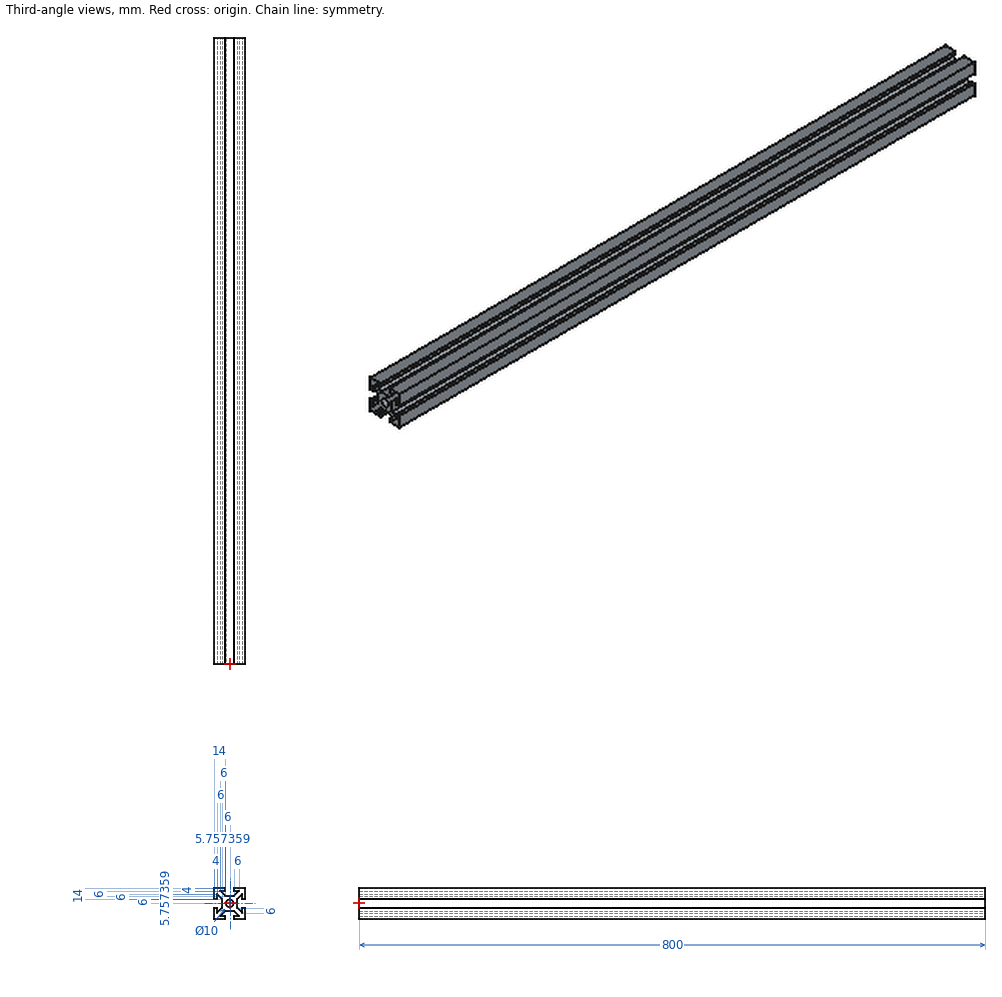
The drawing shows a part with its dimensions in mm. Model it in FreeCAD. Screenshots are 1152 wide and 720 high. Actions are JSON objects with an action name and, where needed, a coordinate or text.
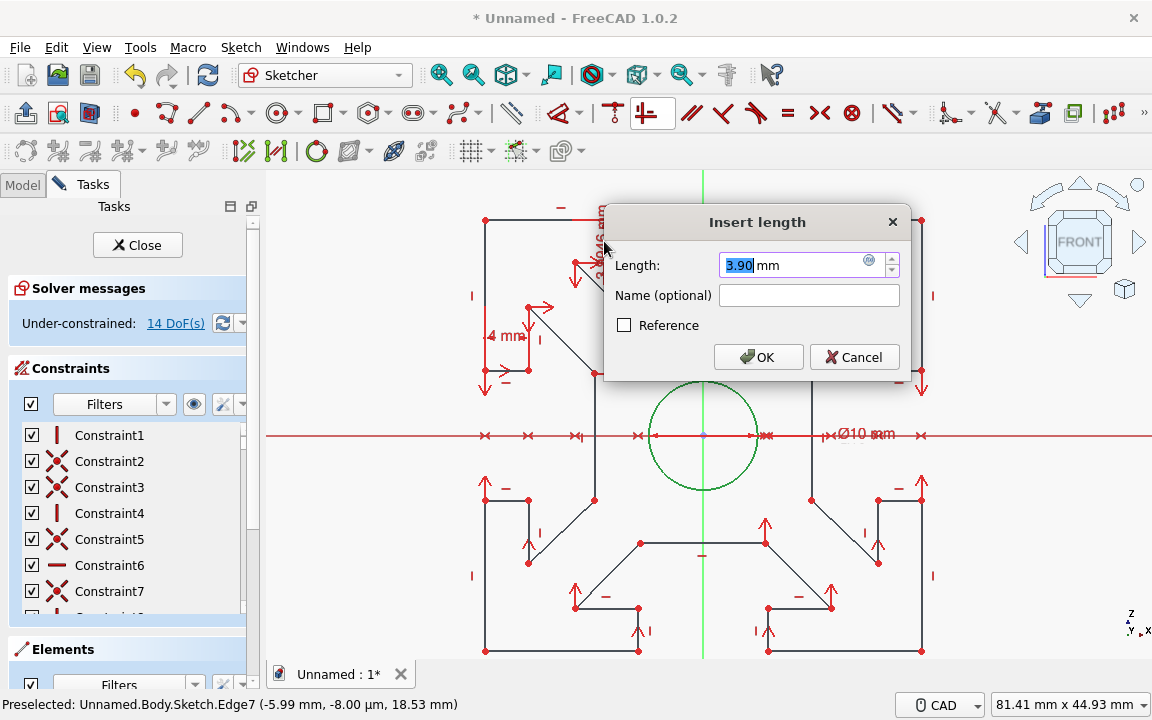
{"action": "type", "text": "4"}
{"action": "key", "text": "Return"}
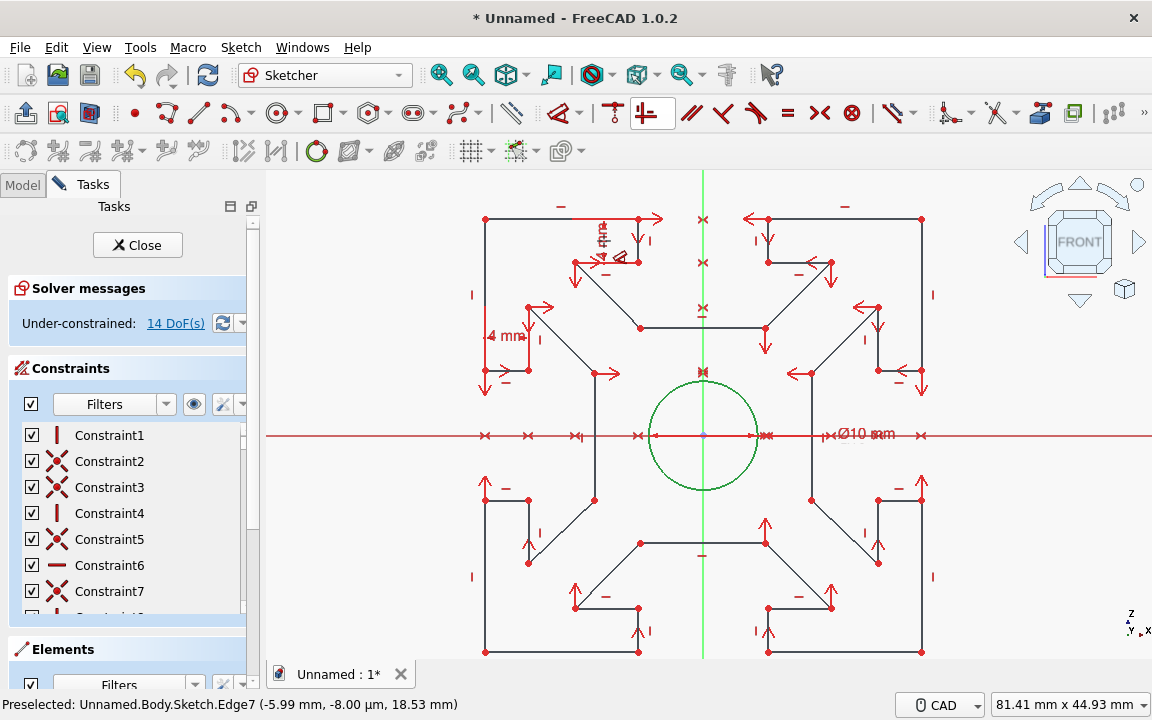
{"action": "left_click", "coordinate": [485, 325]}
{"action": "left_click", "coordinate": [451, 295]}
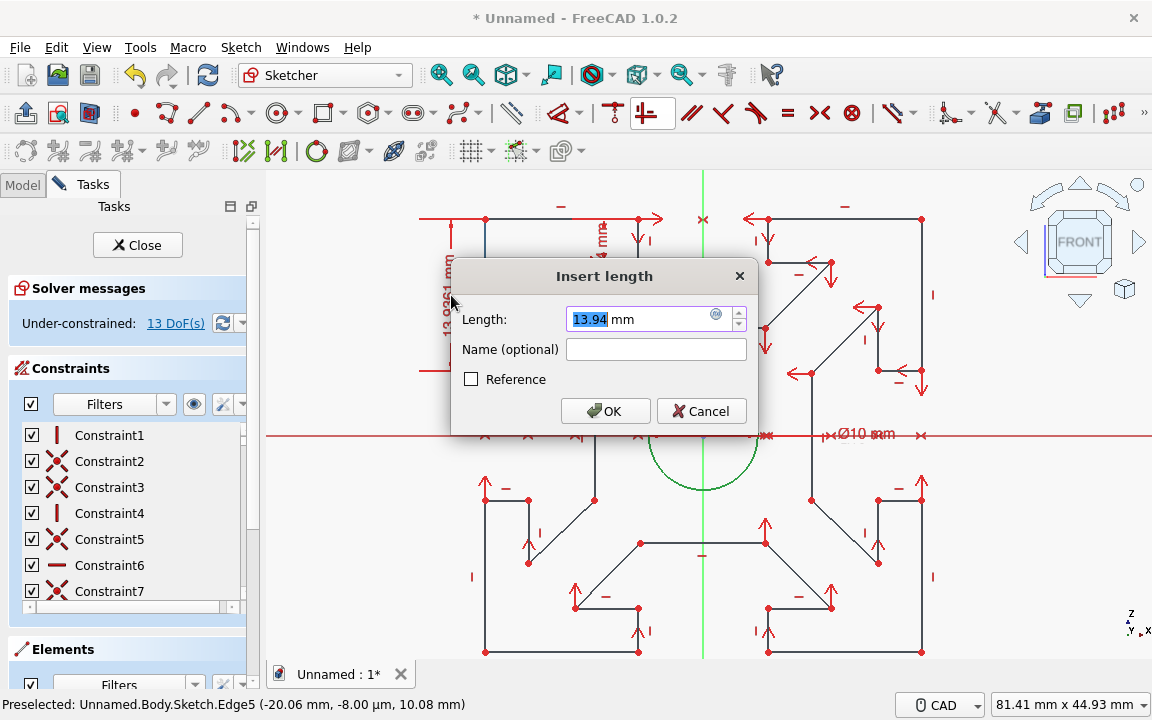
{"action": "type", "text": "14"}
{"action": "key", "text": "Return"}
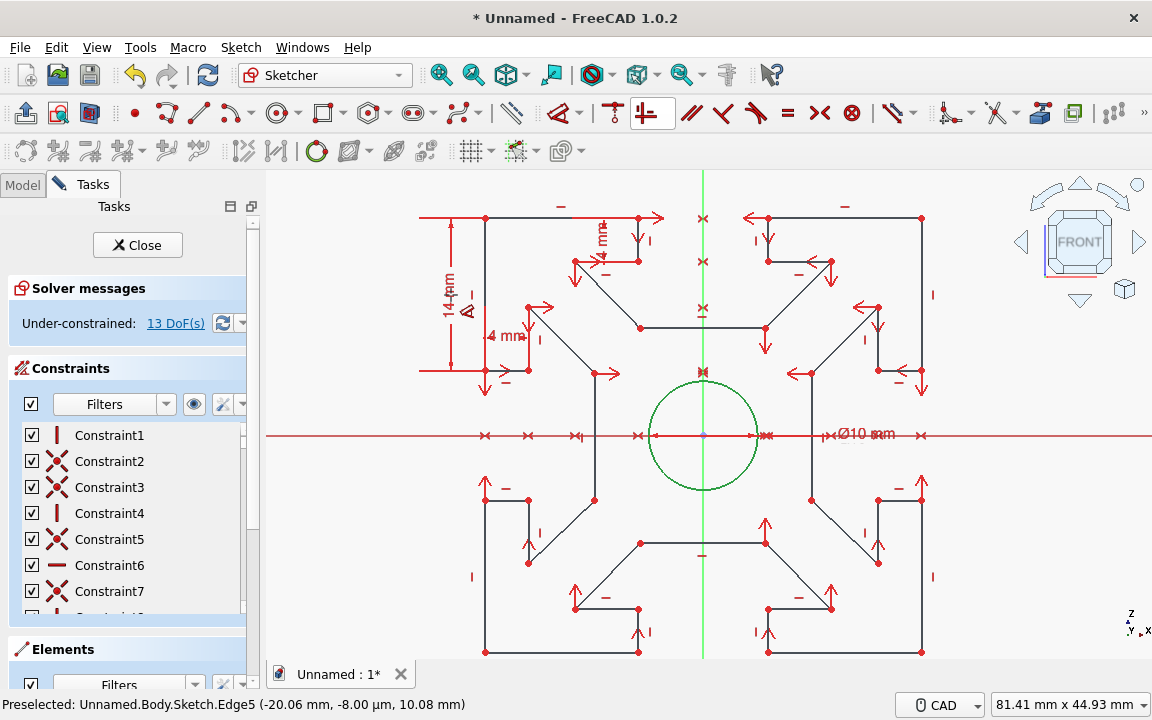
{"action": "left_click", "coordinate": [531, 218]}
{"action": "left_click", "coordinate": [526, 252]}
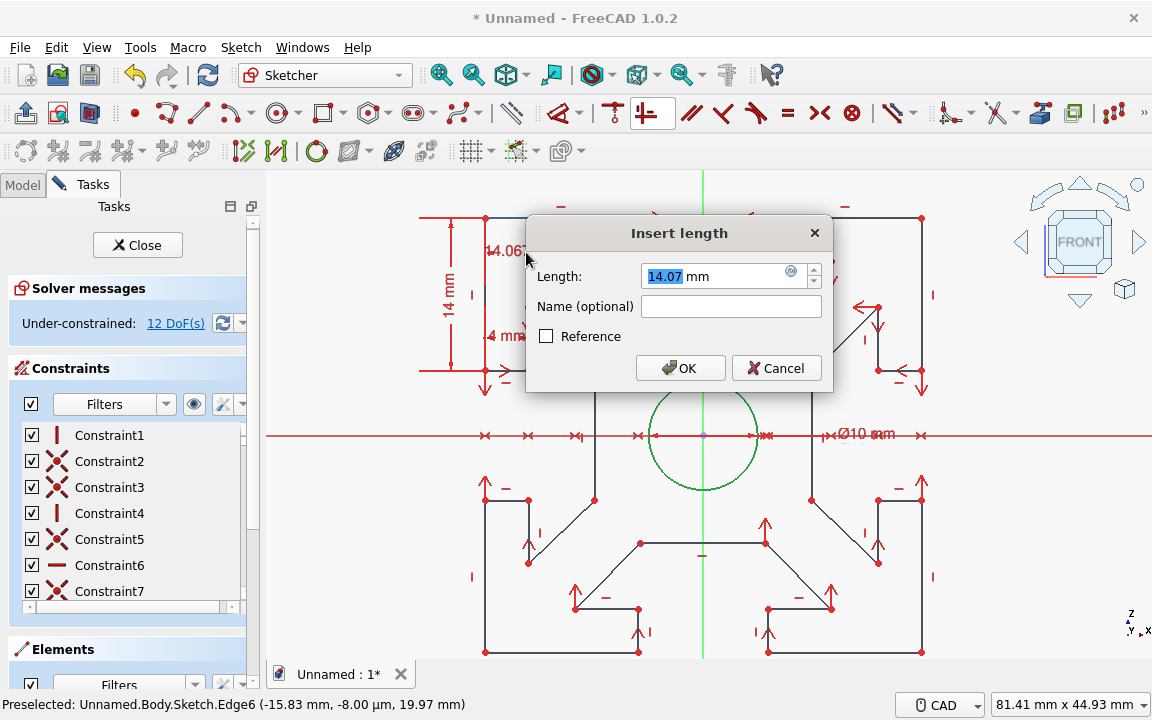
{"action": "type", "text": "14"}
{"action": "key", "text": "Return"}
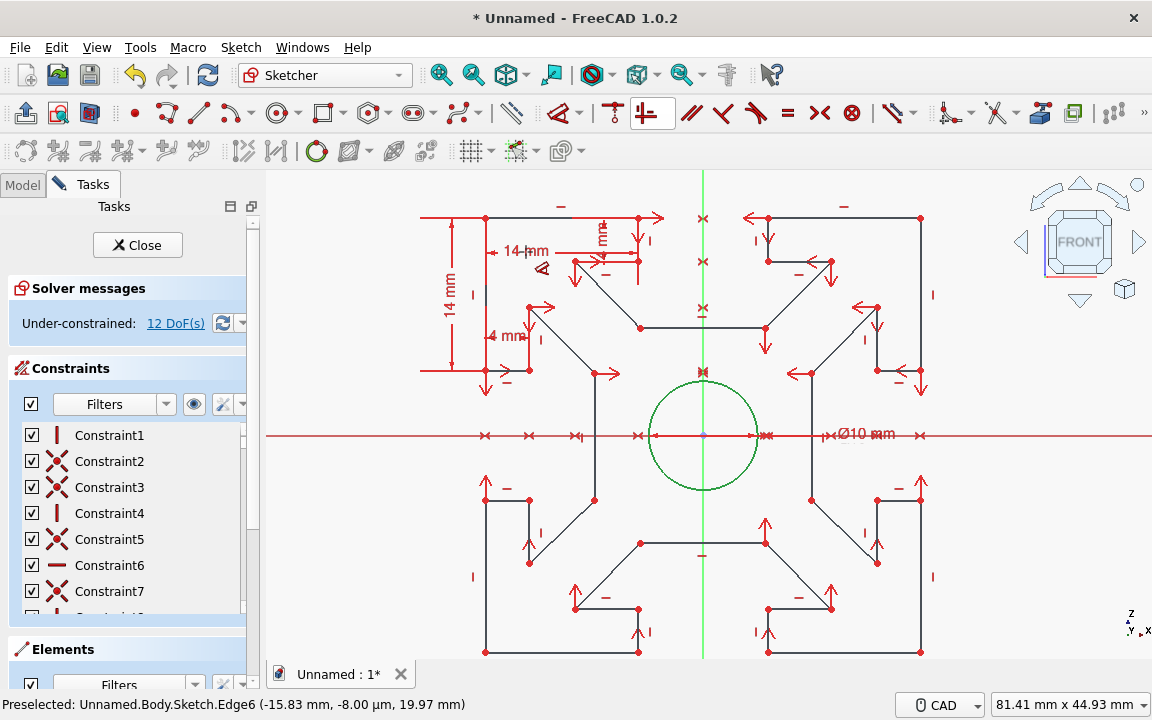
{"action": "left_click", "coordinate": [529, 371]}
{"action": "left_click", "coordinate": [495, 403]}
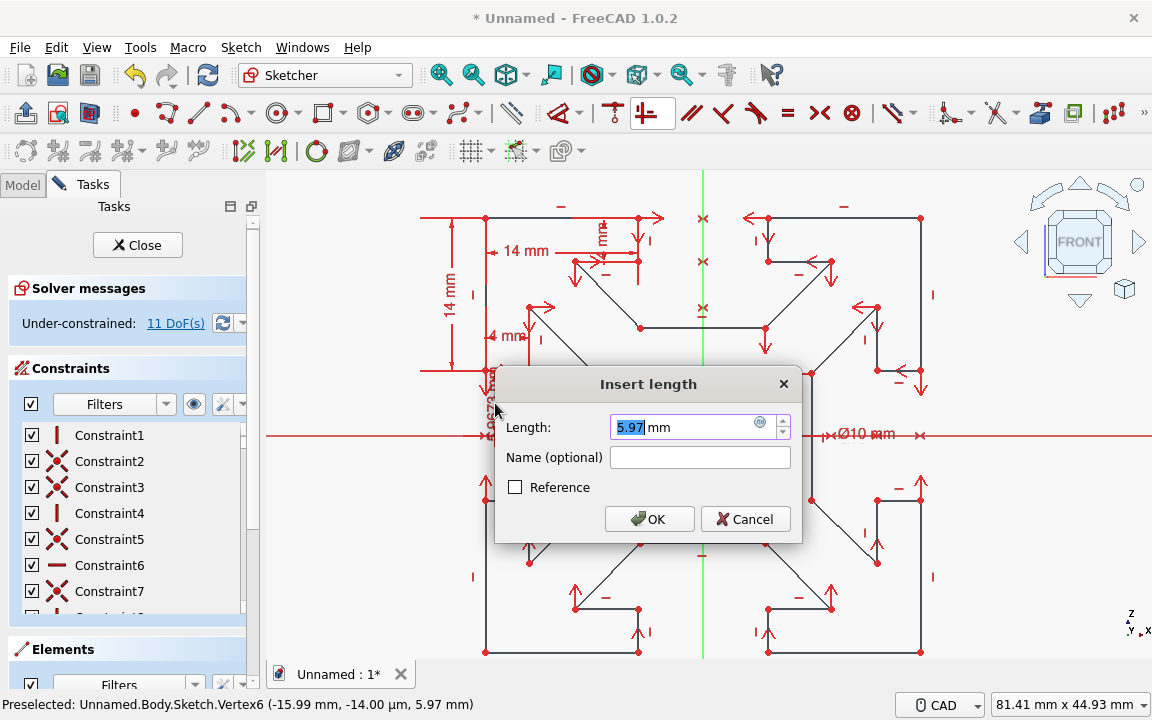
{"action": "type", "text": "6"}
{"action": "key", "text": "Return"}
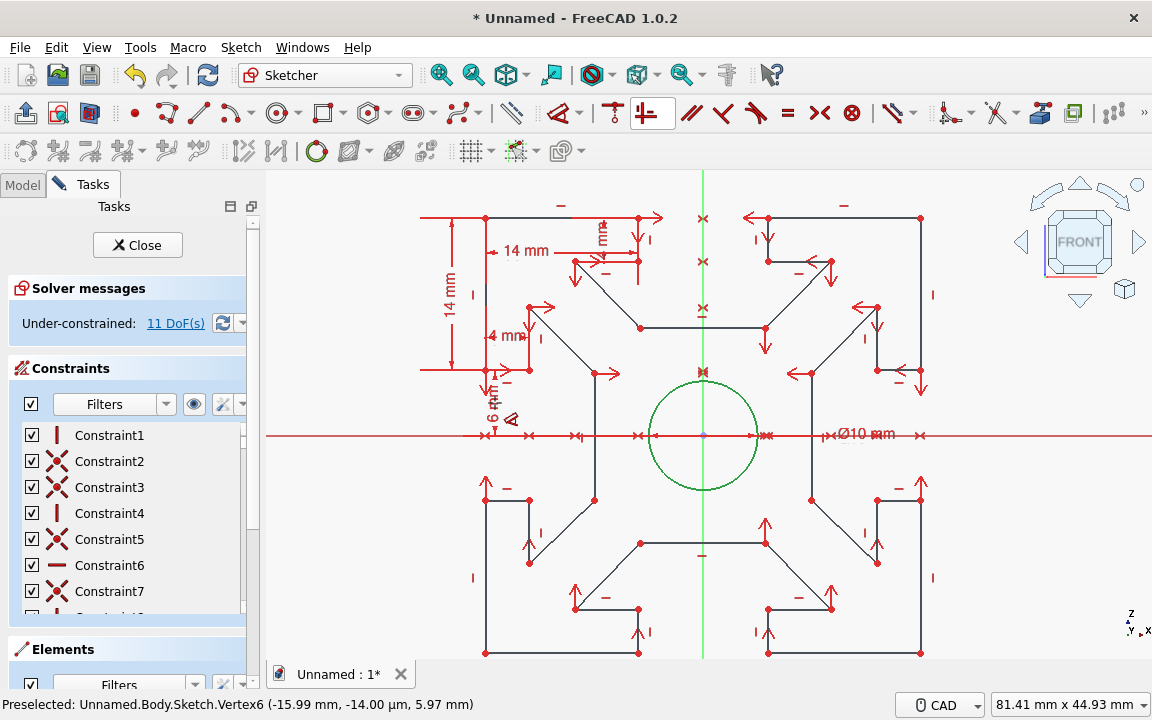
{"action": "left_click", "coordinate": [638, 218]}
{"action": "left_click", "coordinate": [686, 470]}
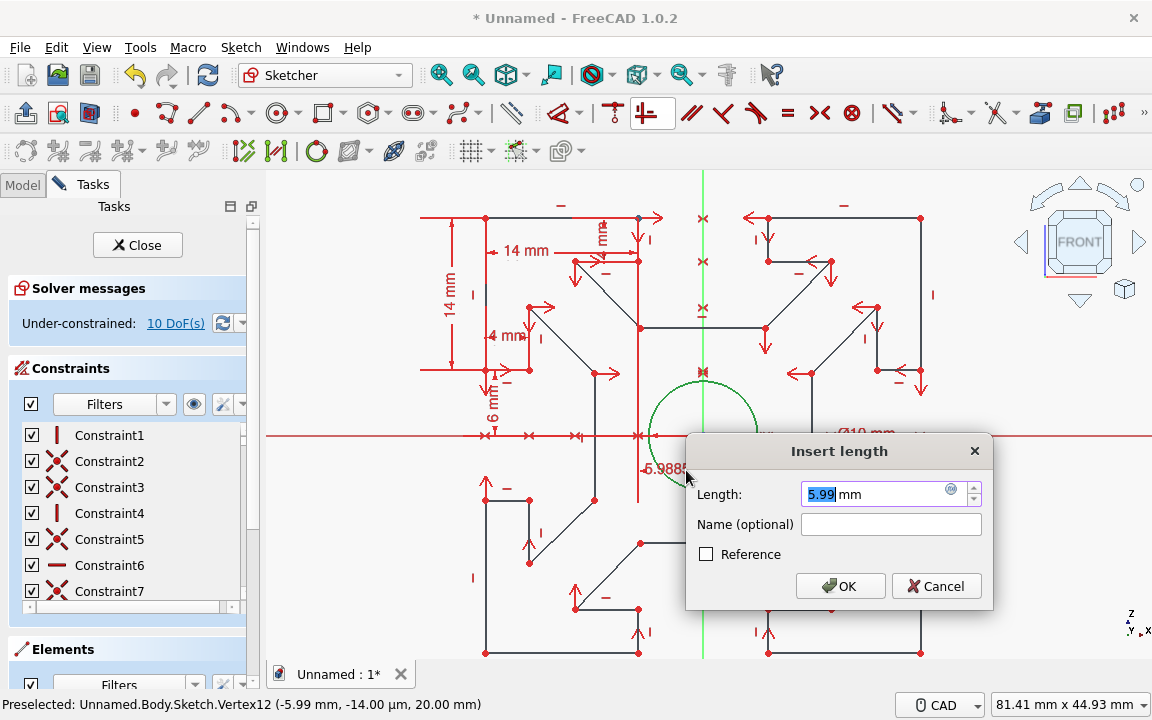
{"action": "type", "text": "6"}
{"action": "key", "text": "Return"}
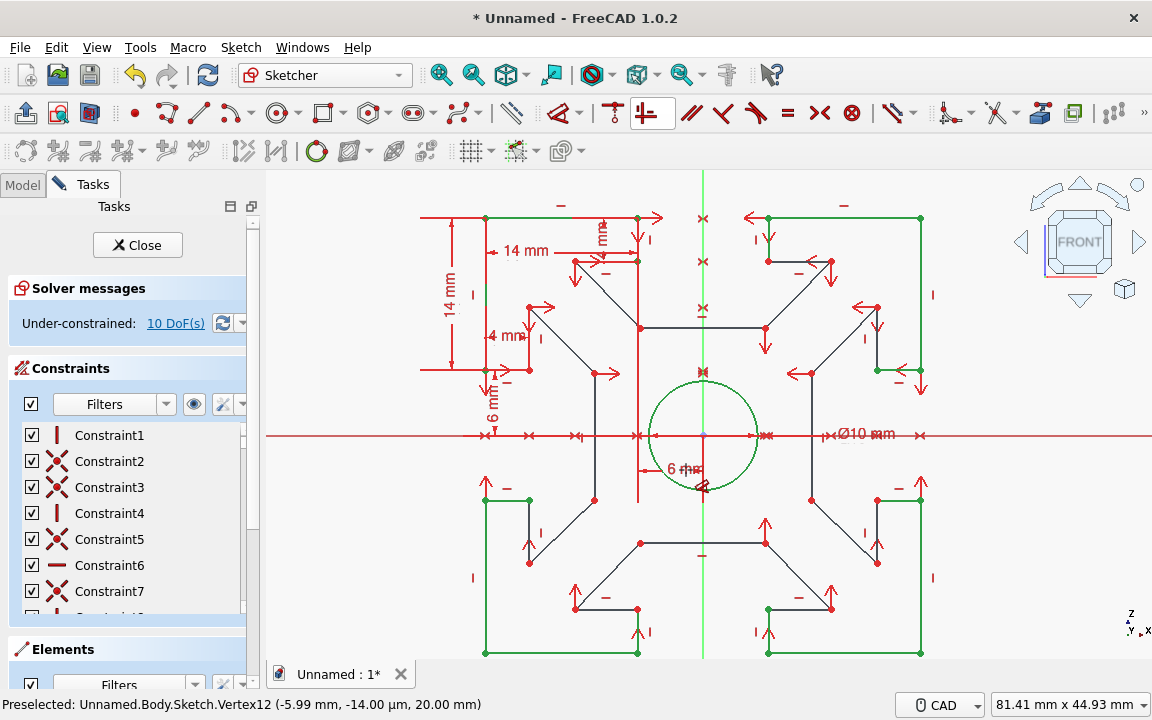
{"action": "left_click", "coordinate": [575, 354]}
{"action": "left_click", "coordinate": [562, 273]}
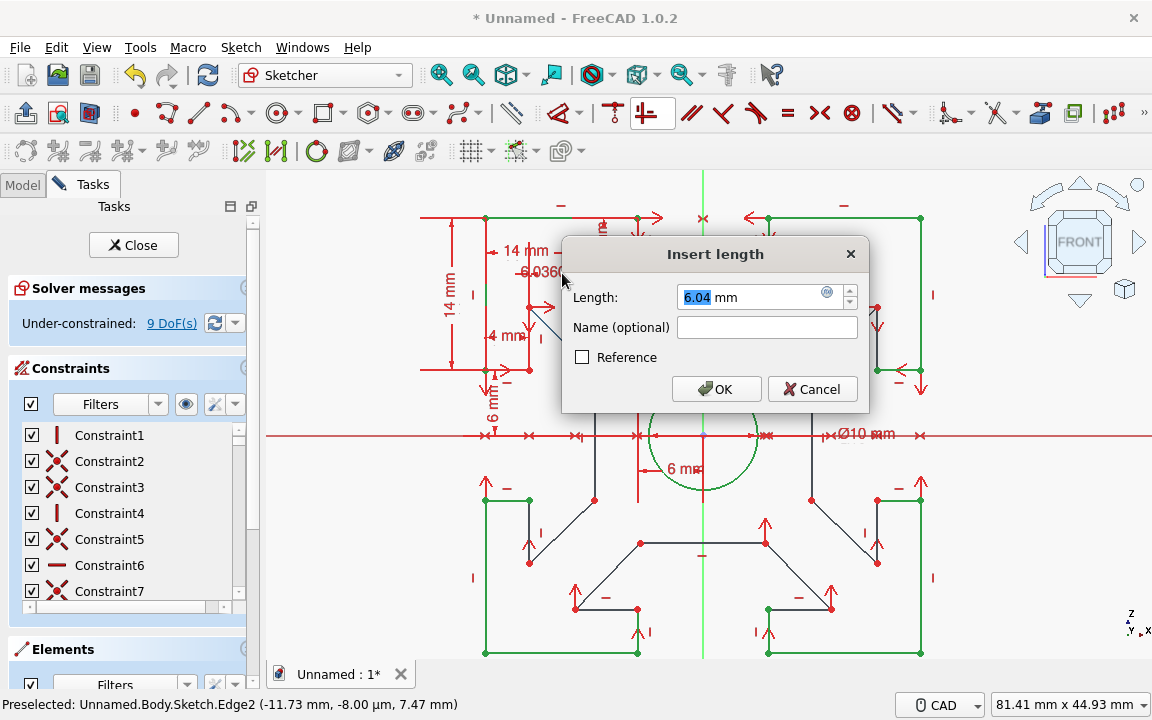
{"action": "type", "text": "6"}
{"action": "key", "text": "Return"}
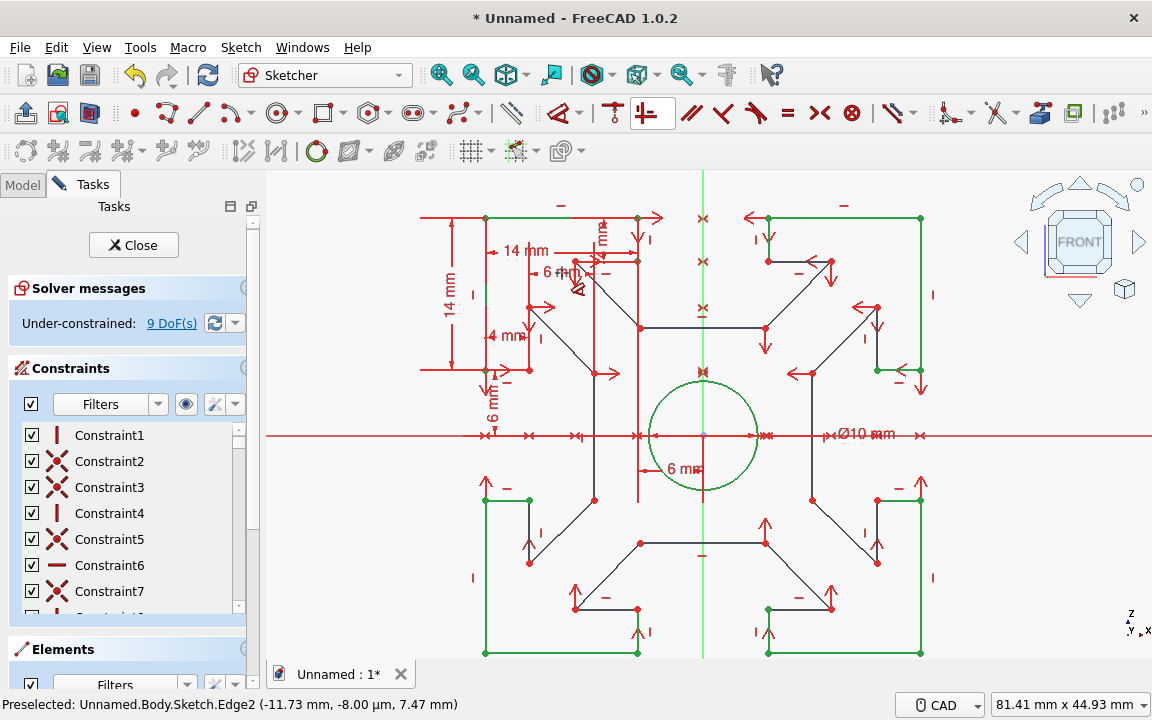
{"action": "left_click", "coordinate": [575, 354]}
{"action": "left_click", "coordinate": [628, 341]}